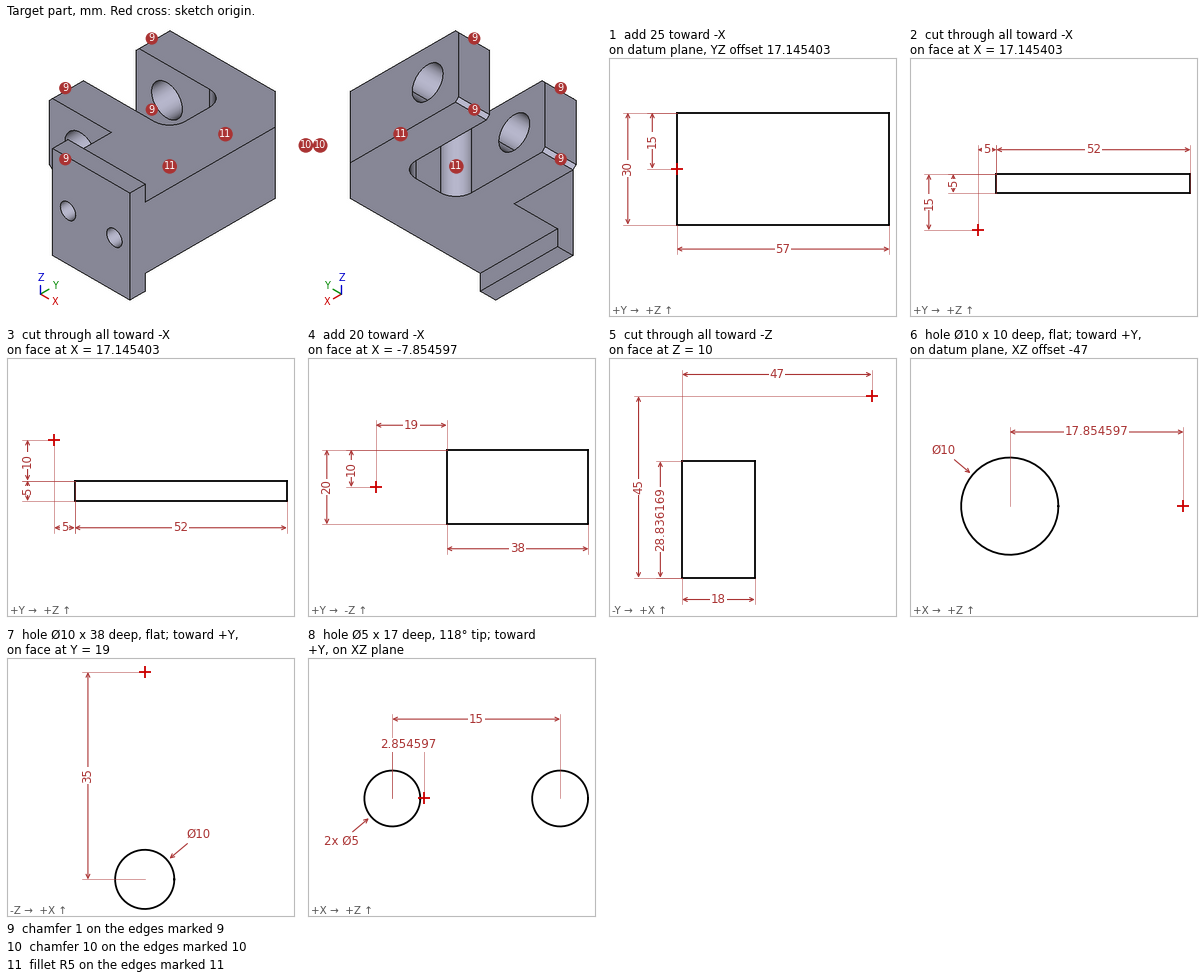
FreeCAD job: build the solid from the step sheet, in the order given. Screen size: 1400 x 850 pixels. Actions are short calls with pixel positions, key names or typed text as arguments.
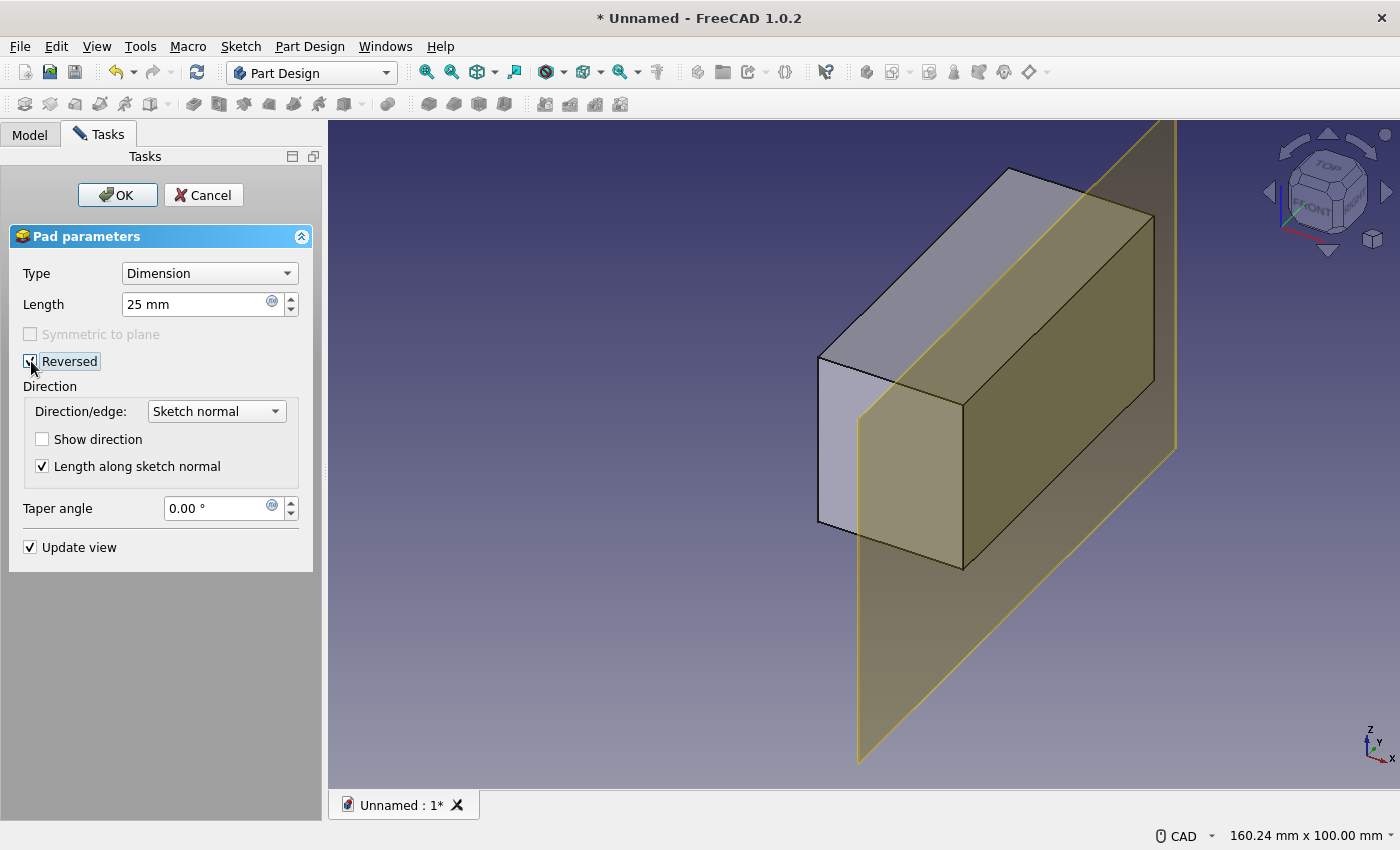
click(118, 195)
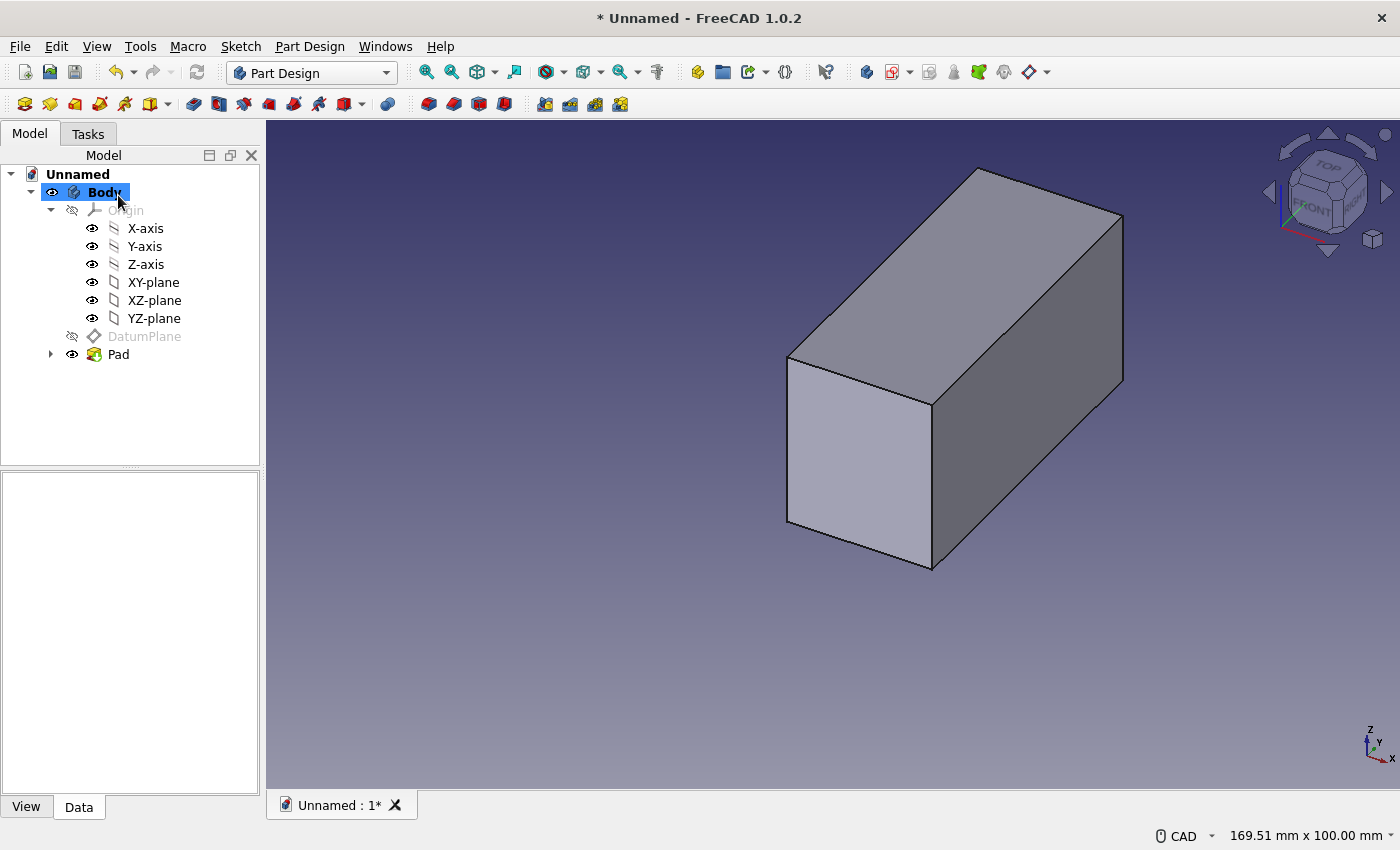
click(1055, 365)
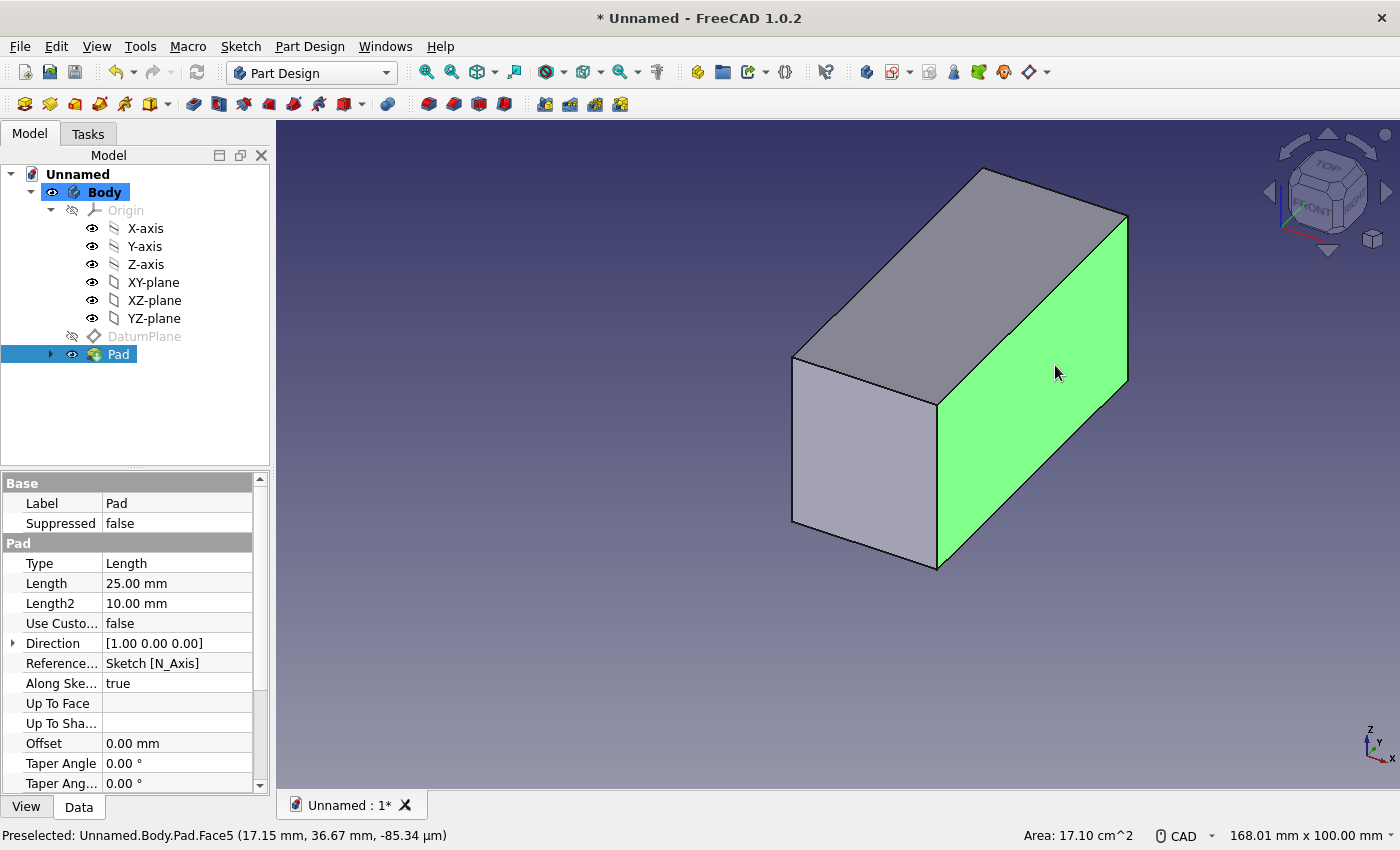
click(892, 72)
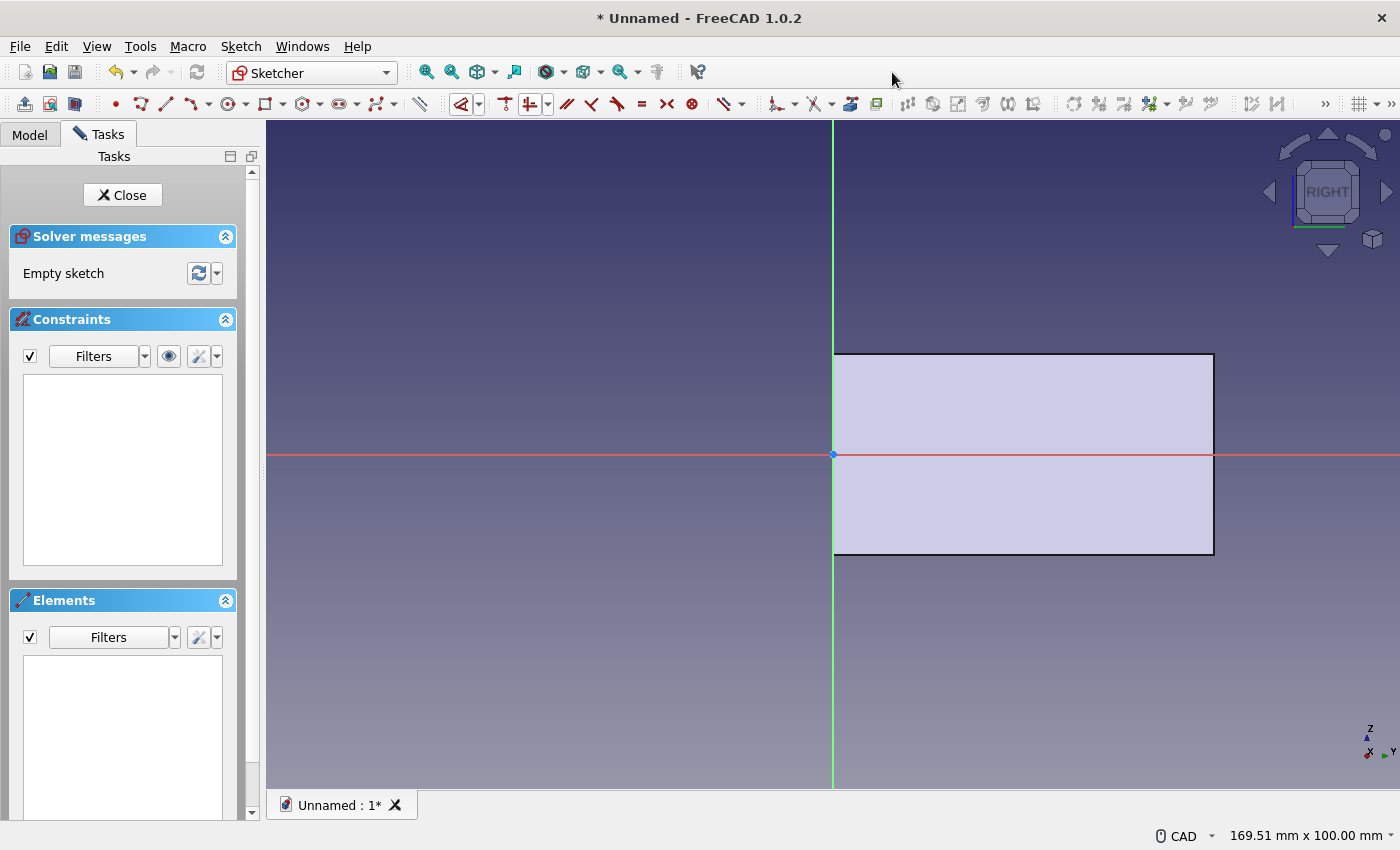
scroll(1235, 343, up, 3)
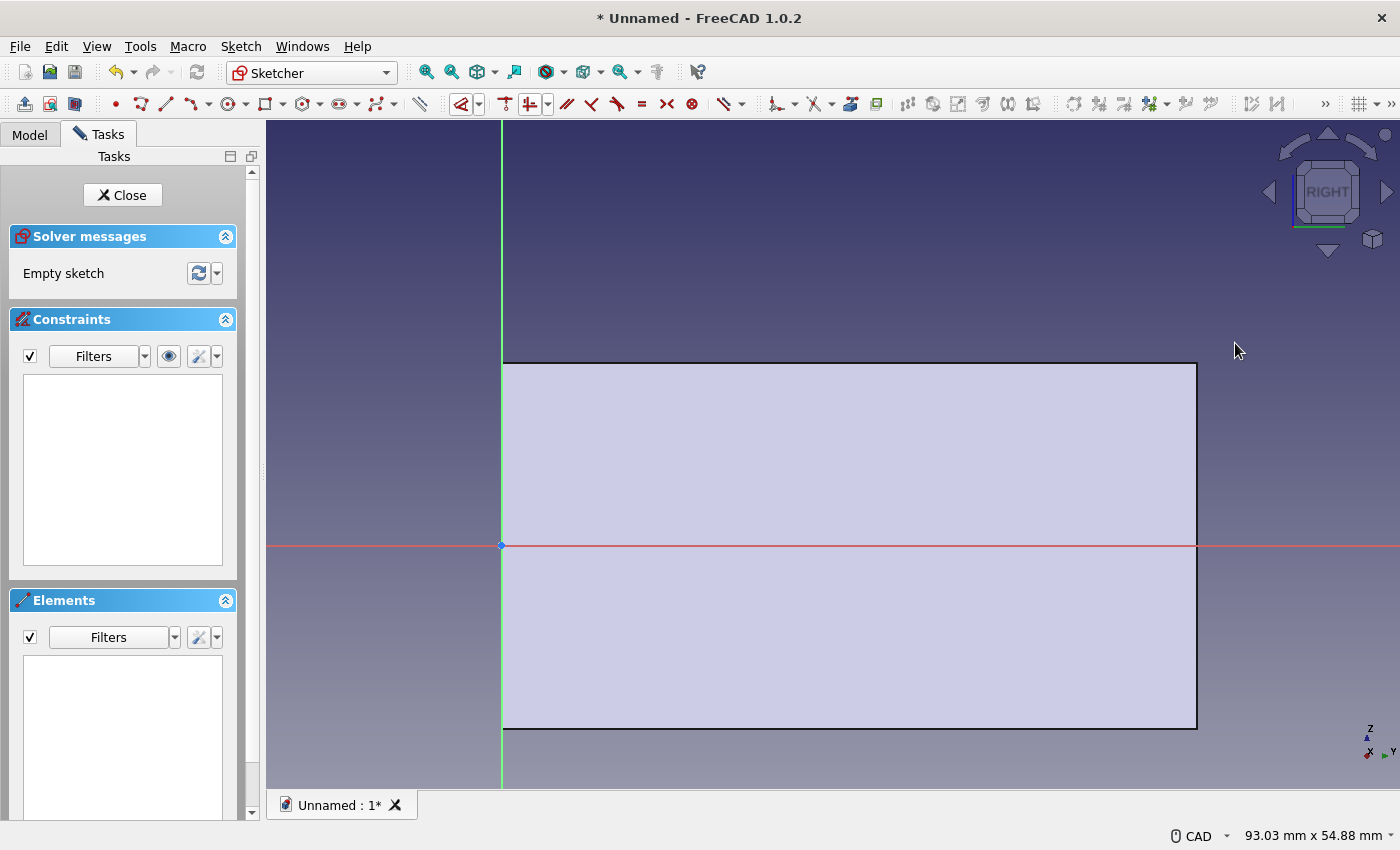
click(264, 104)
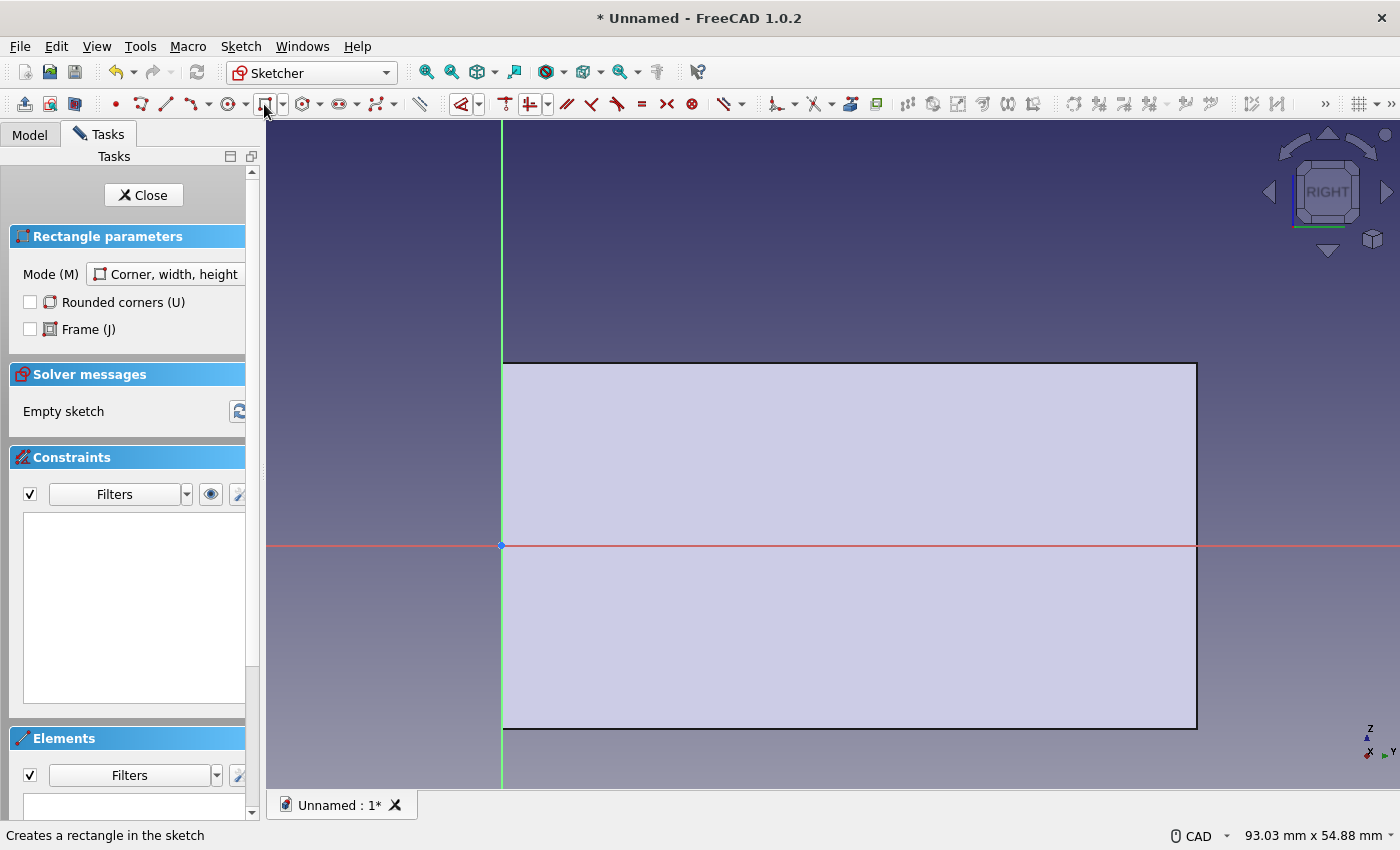
click(563, 363)
click(1197, 424)
key(Escape)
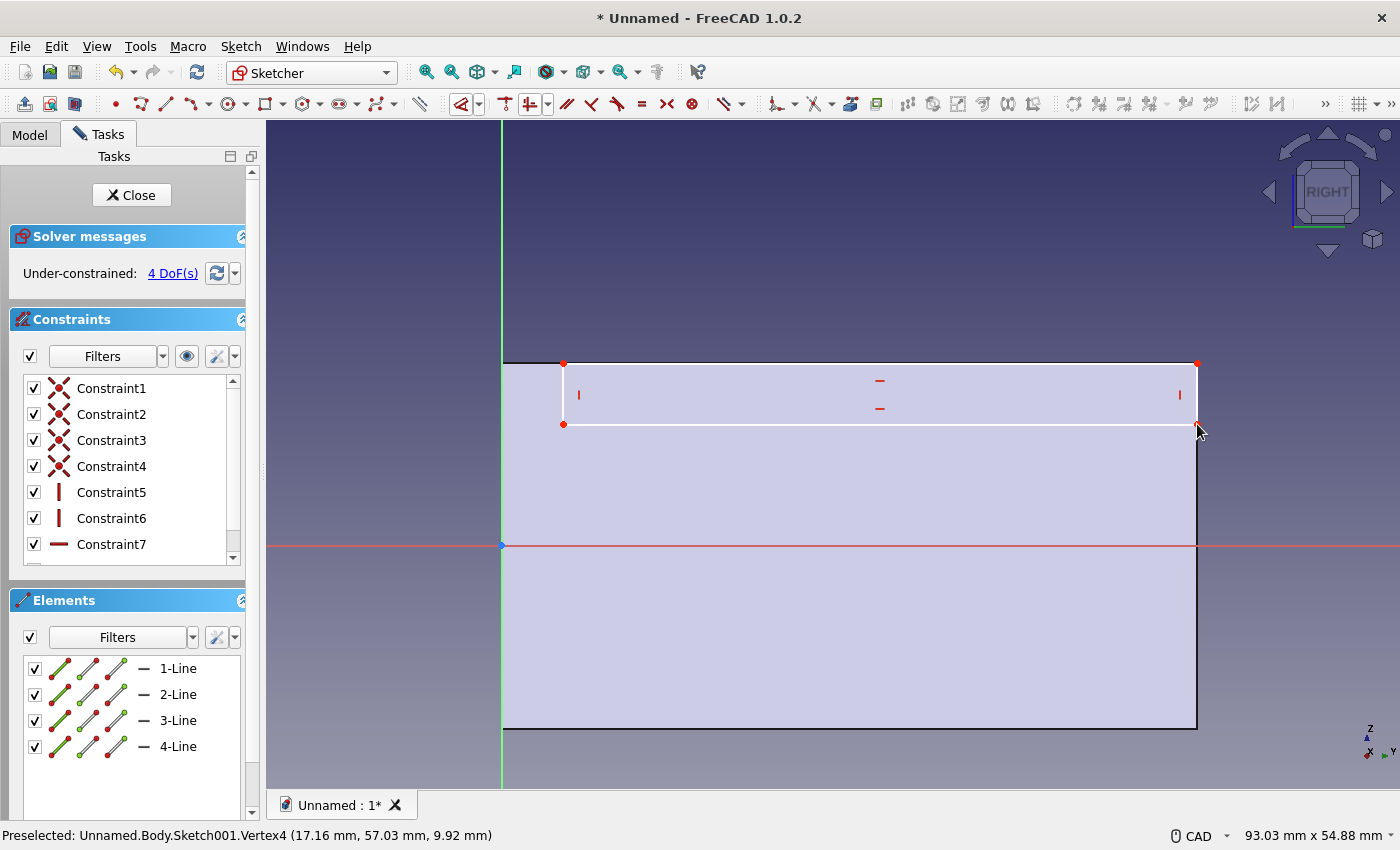
click(460, 104)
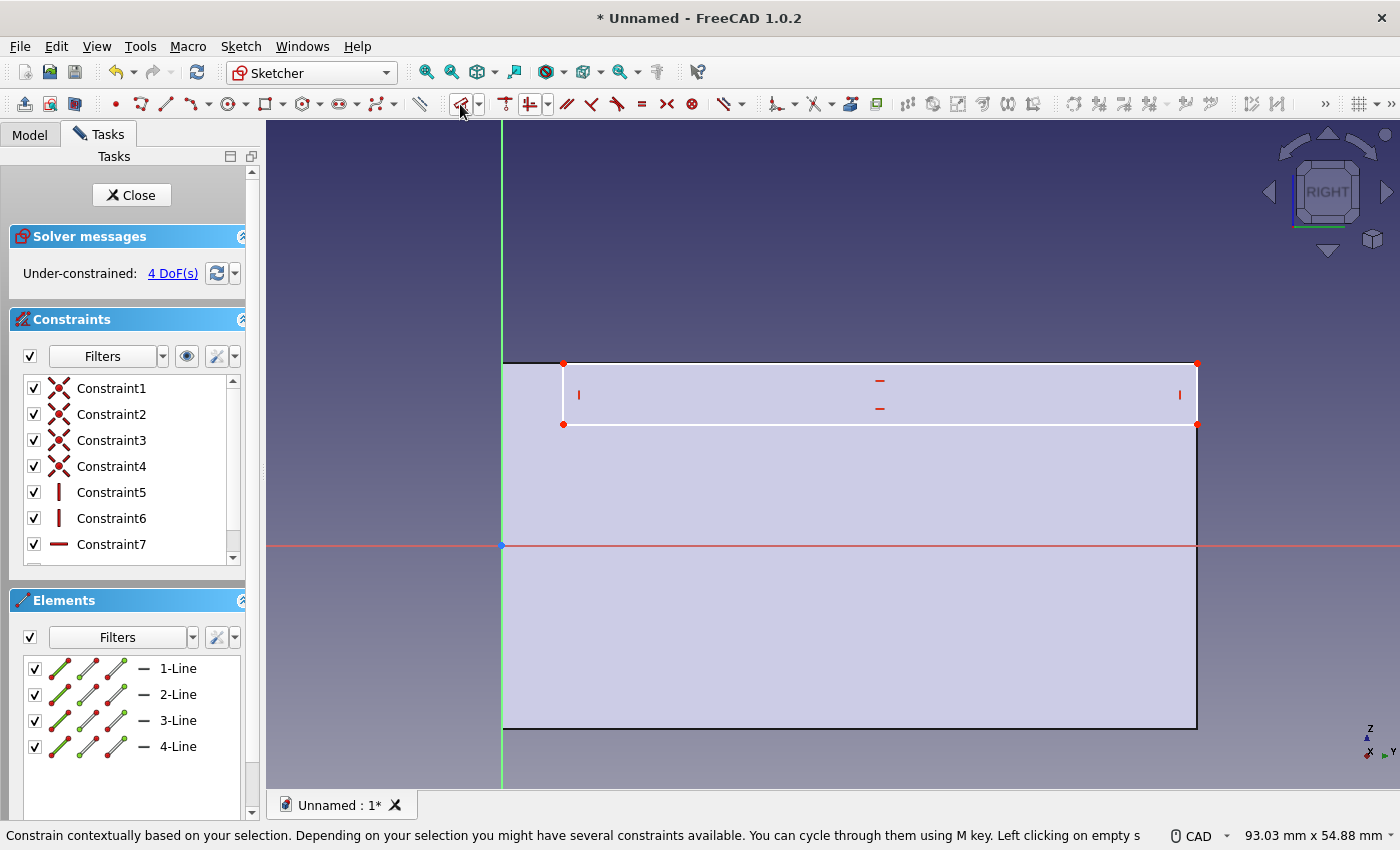
click(563, 382)
click(529, 394)